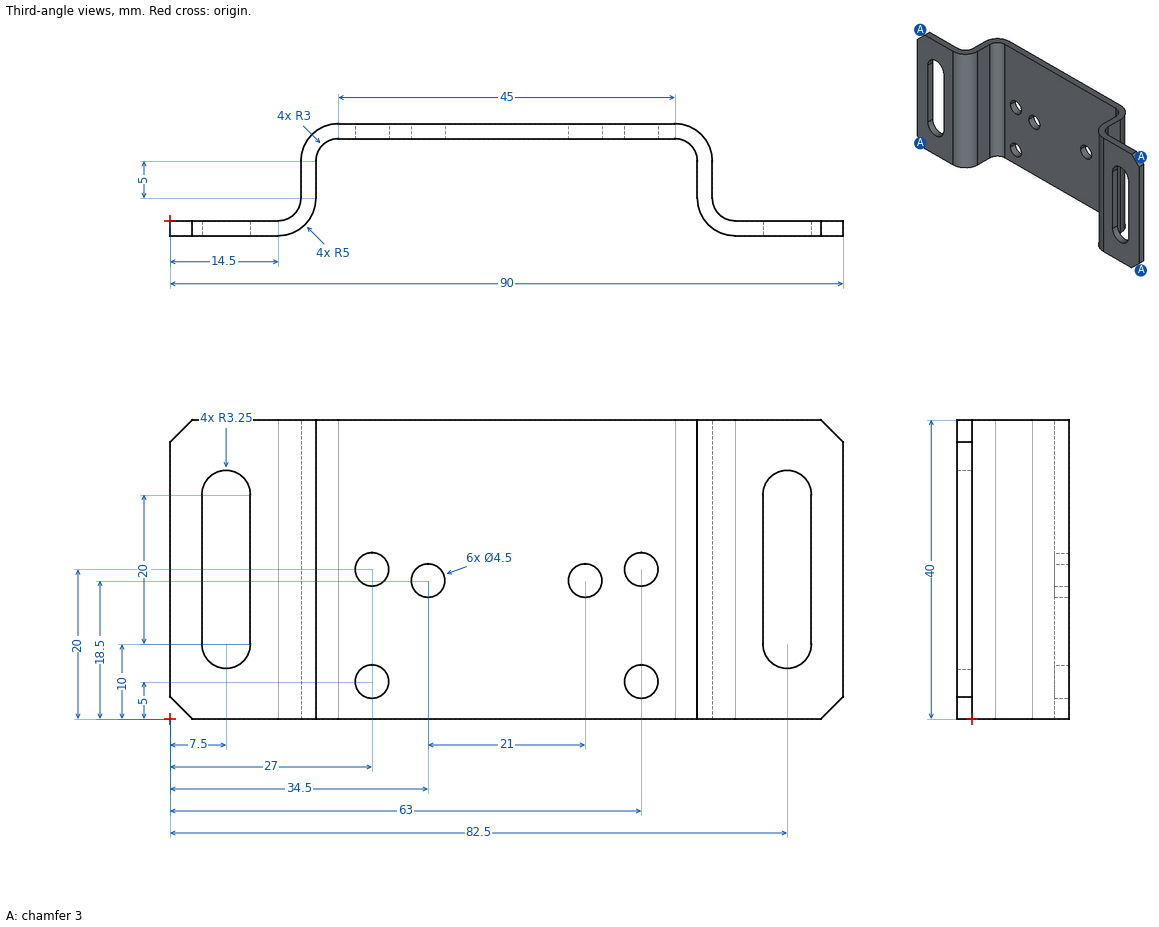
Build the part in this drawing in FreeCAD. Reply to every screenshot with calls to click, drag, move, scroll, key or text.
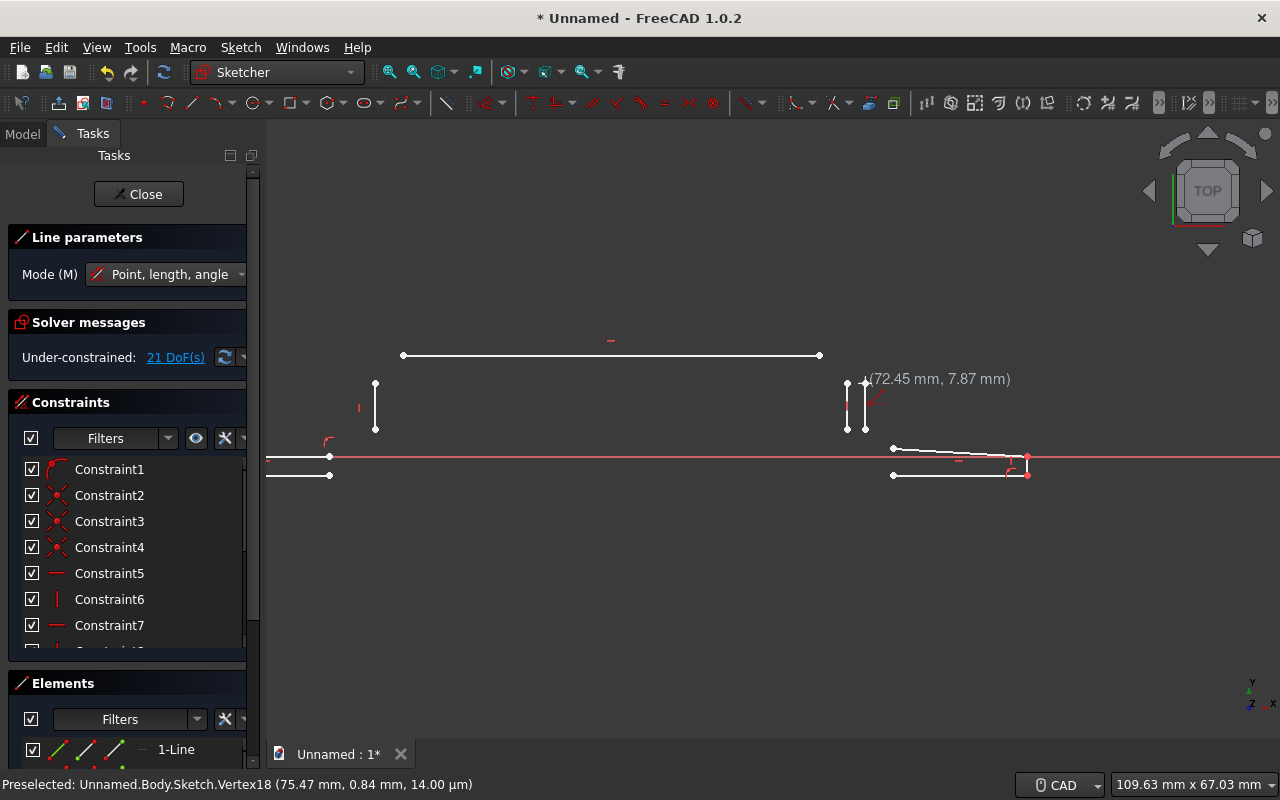
click(819, 337)
click(403, 337)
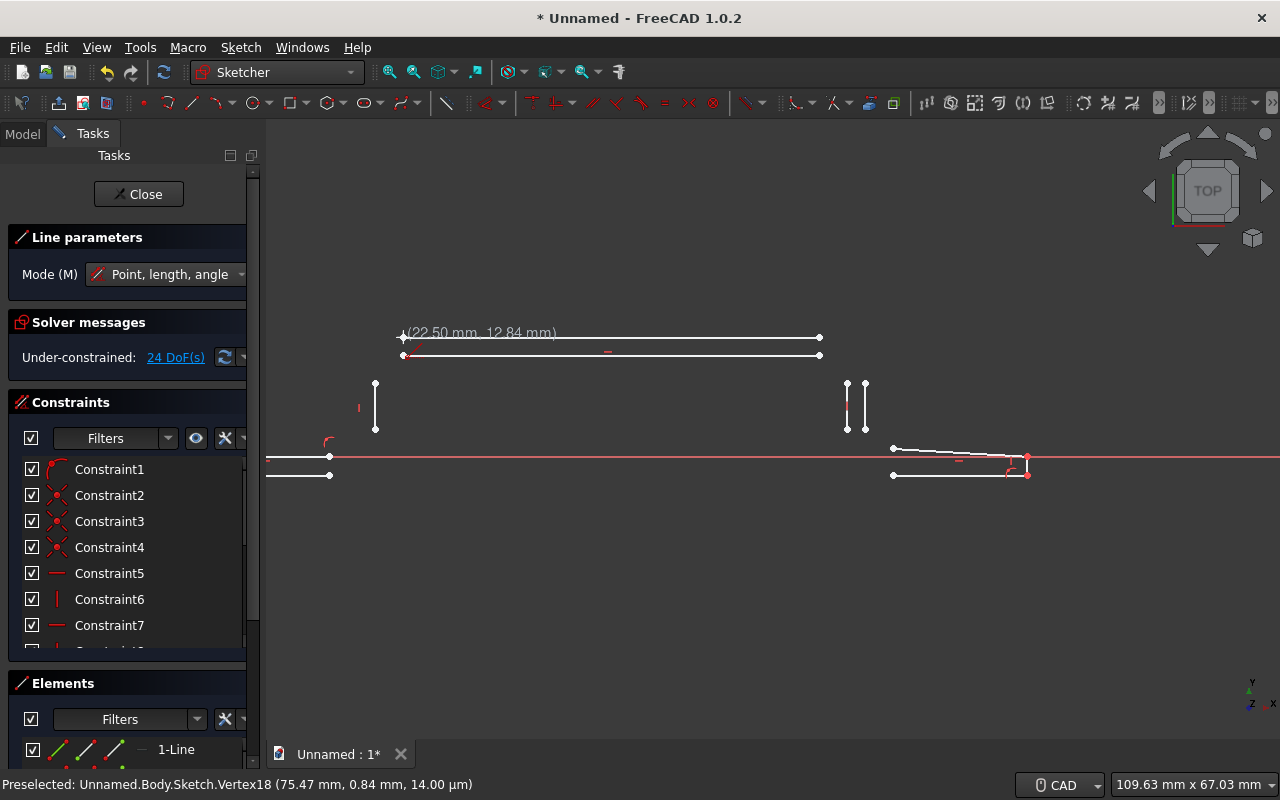
click(357, 383)
click(357, 429)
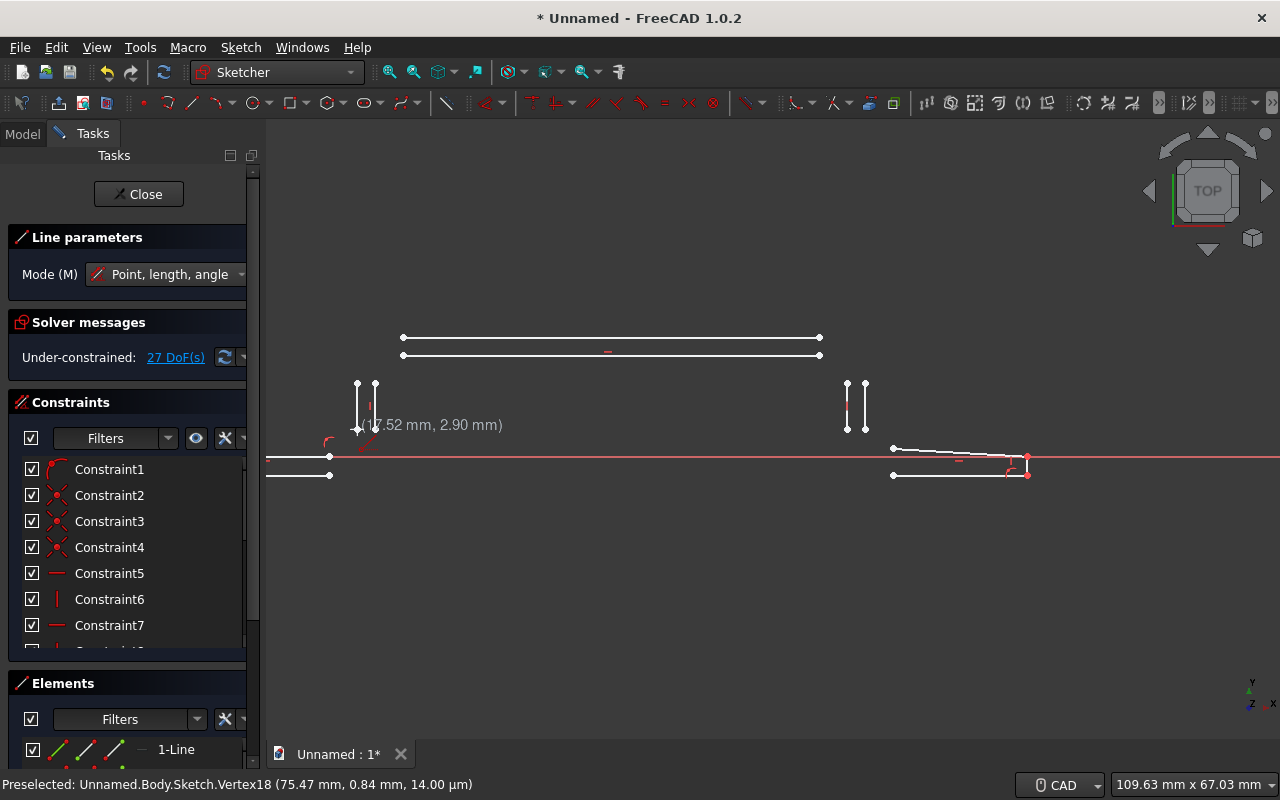
key(g)
key(3)
key(a)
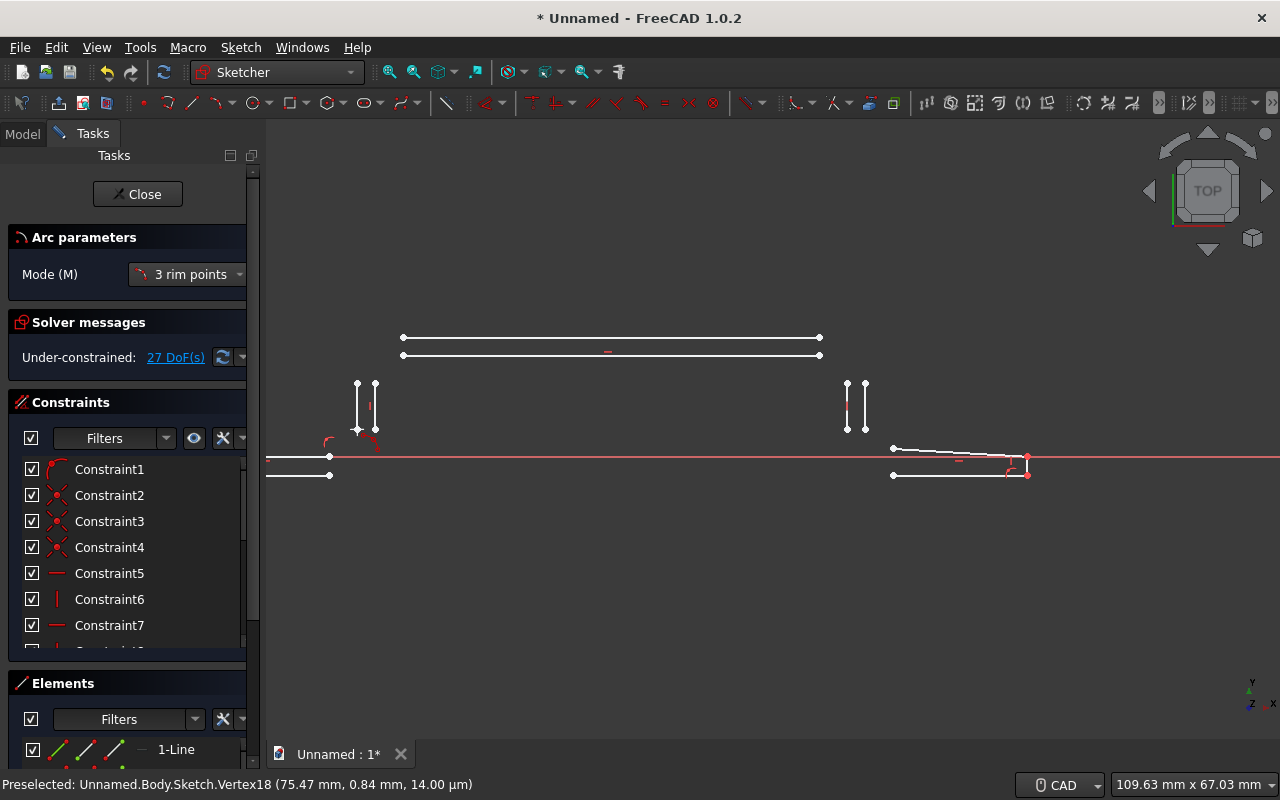
click(329, 476)
click(375, 430)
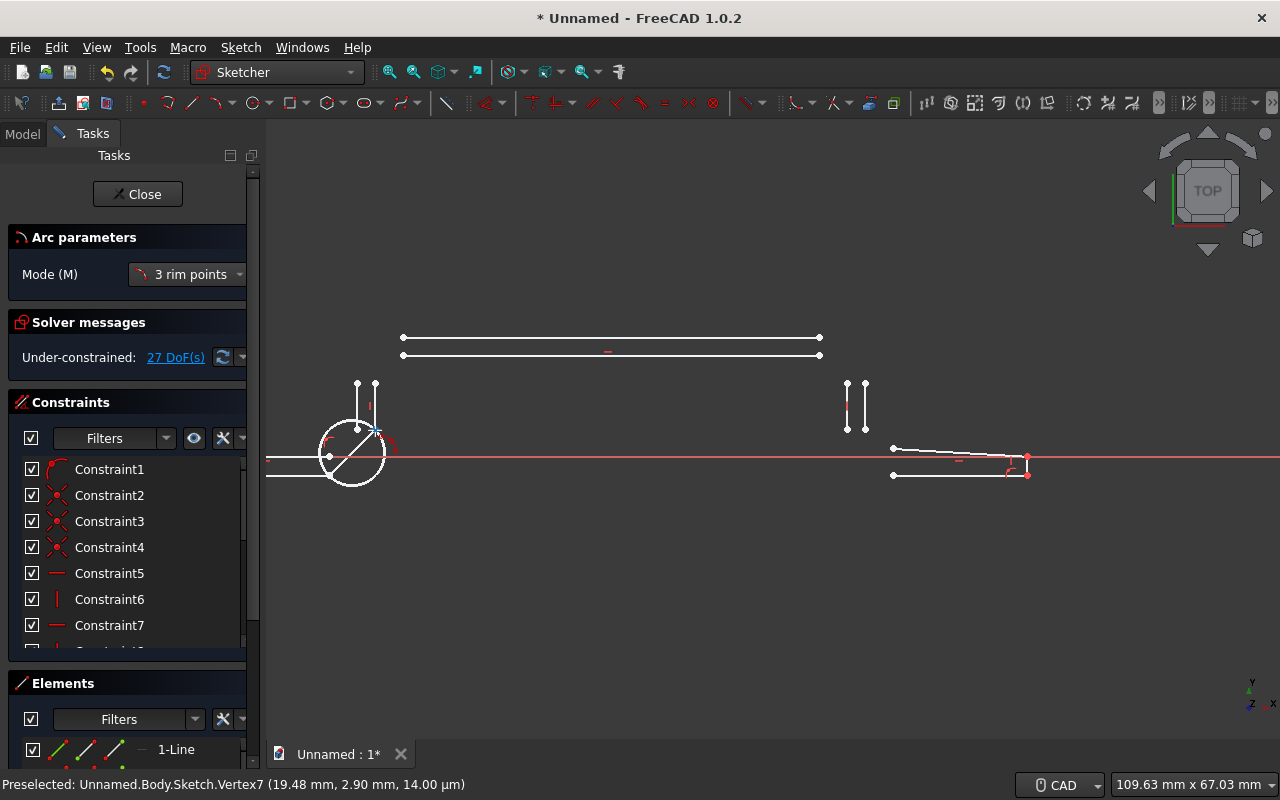
scroll(350, 470, up, 2)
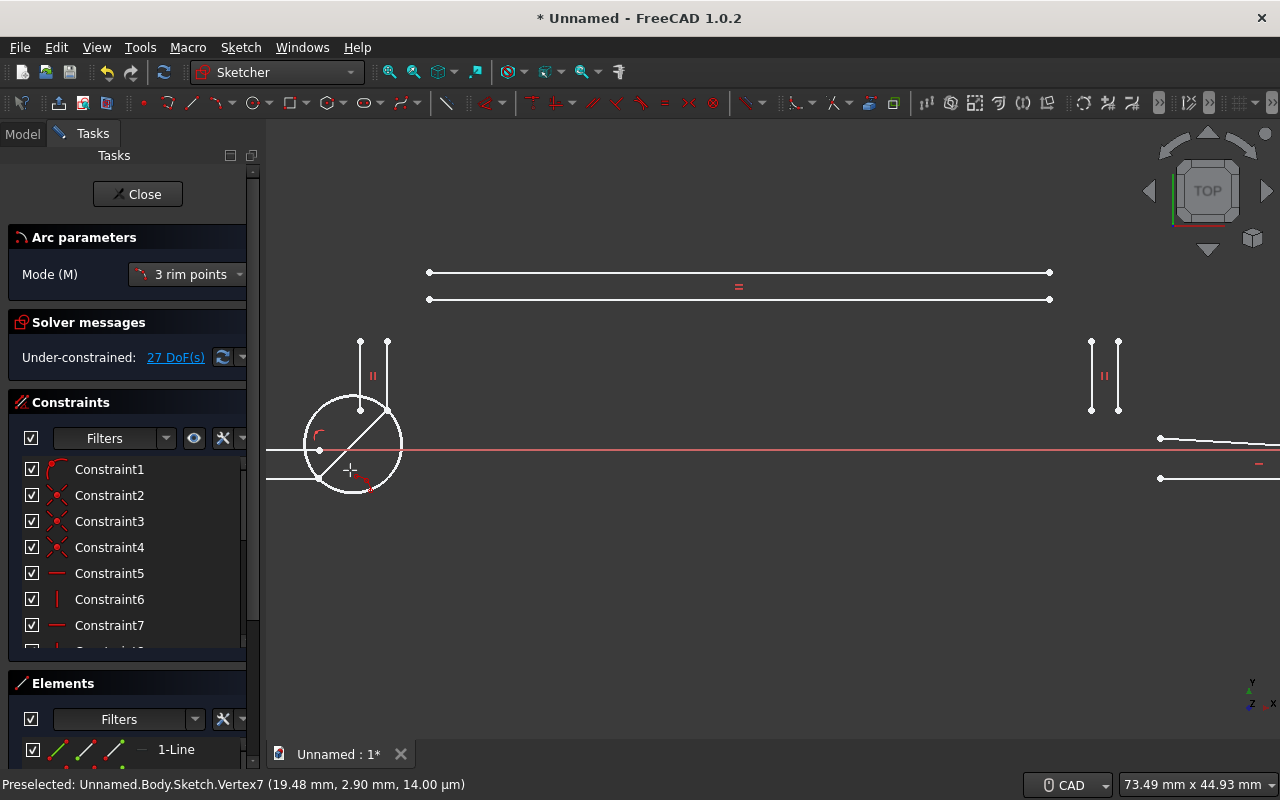
click(350, 470)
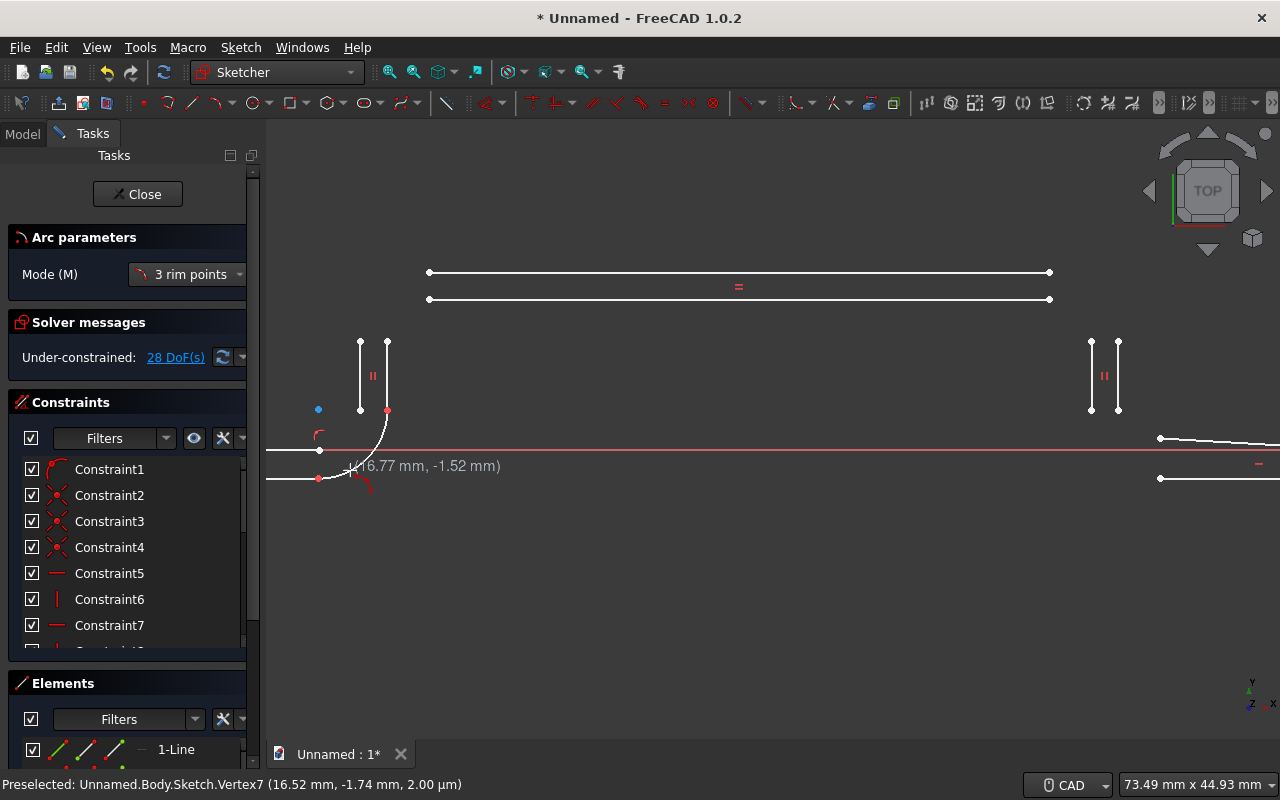
click(387, 341)
click(429, 300)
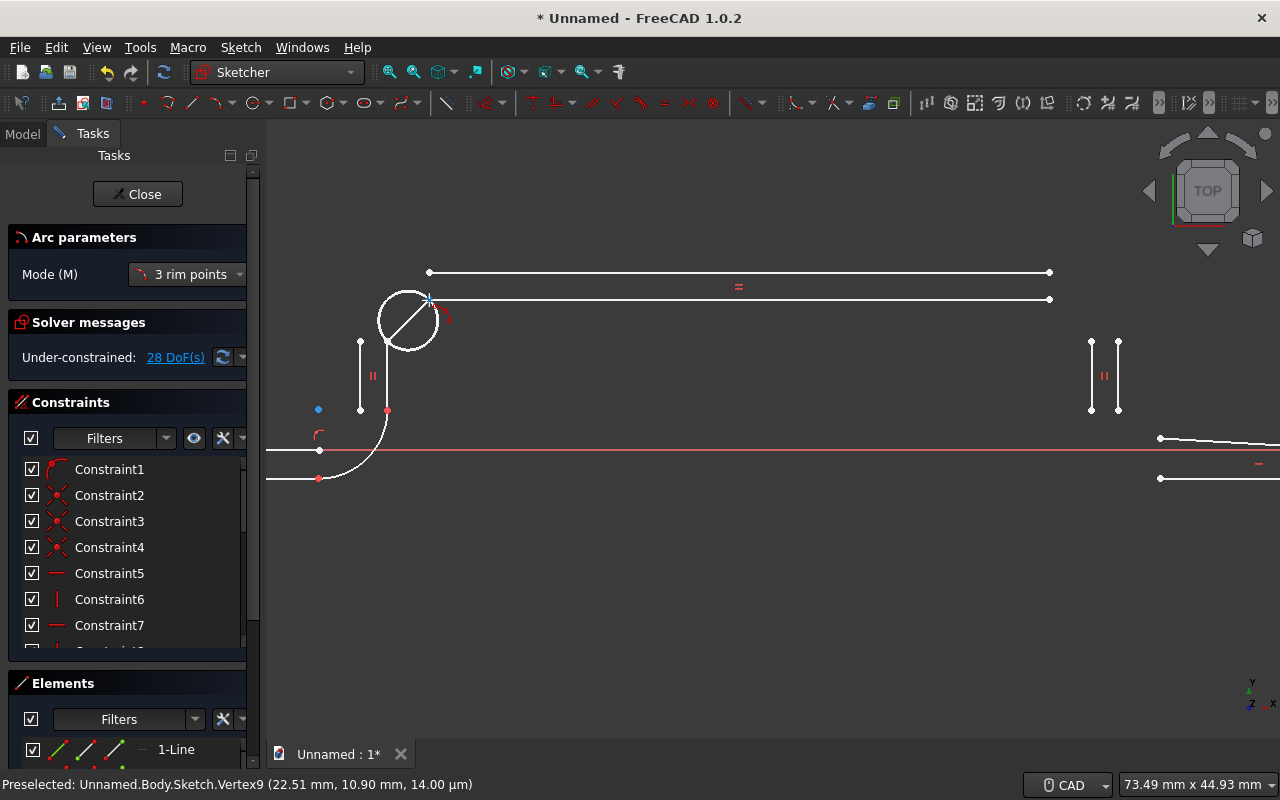
scroll(400, 310, up, 2)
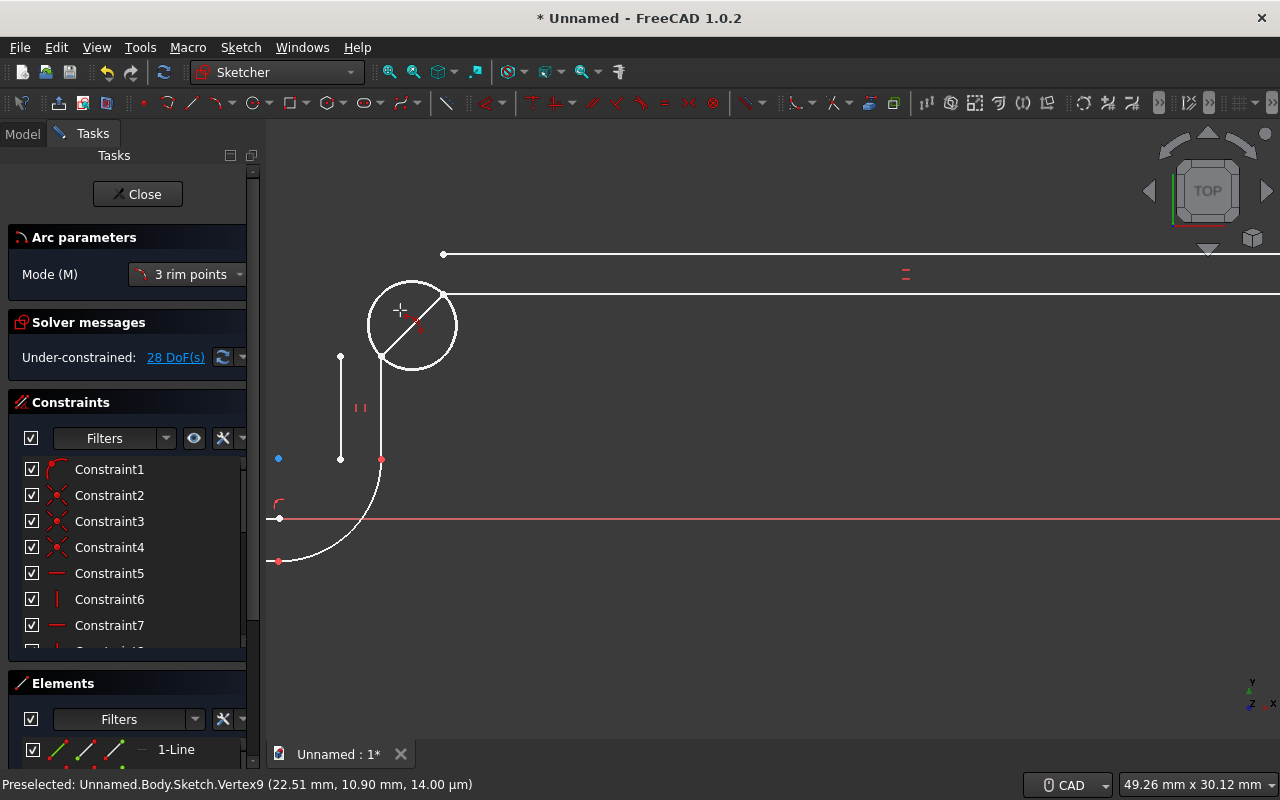
click(400, 310)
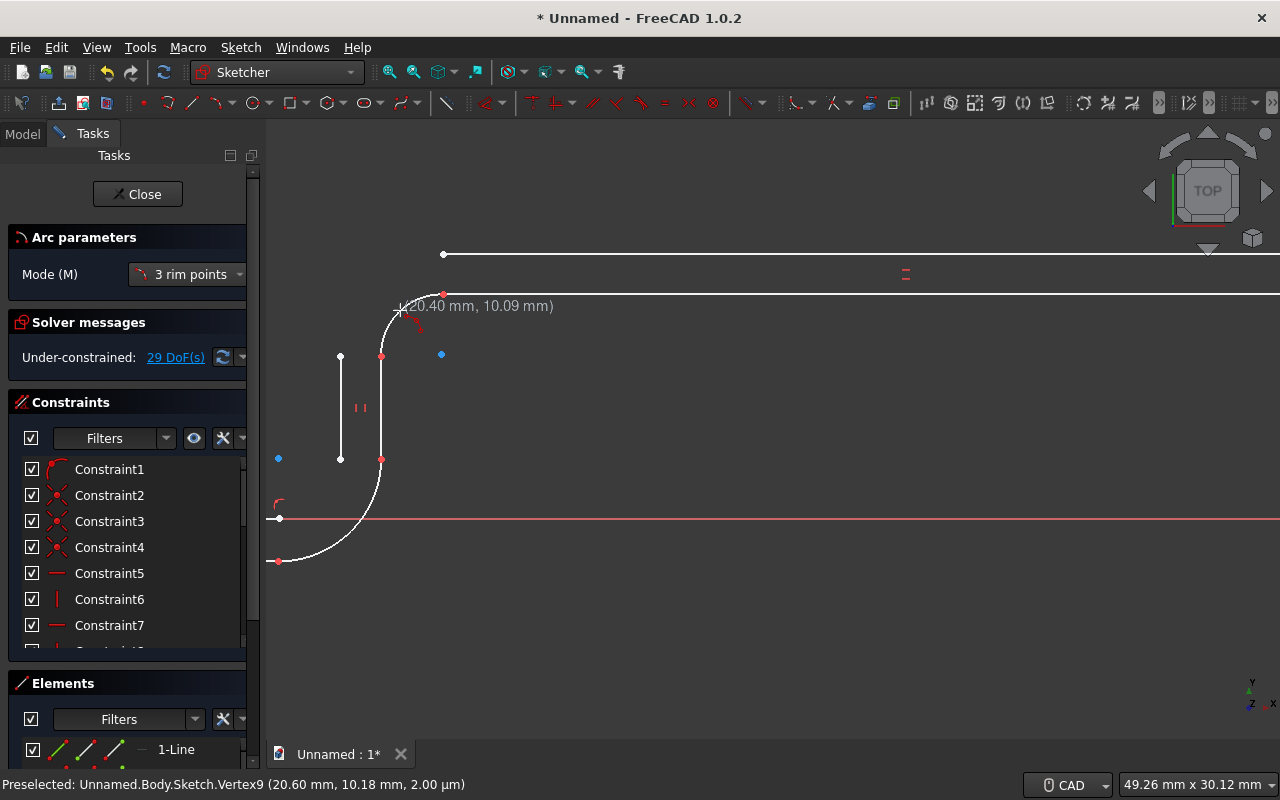
scroll(617, 439, down, 6)